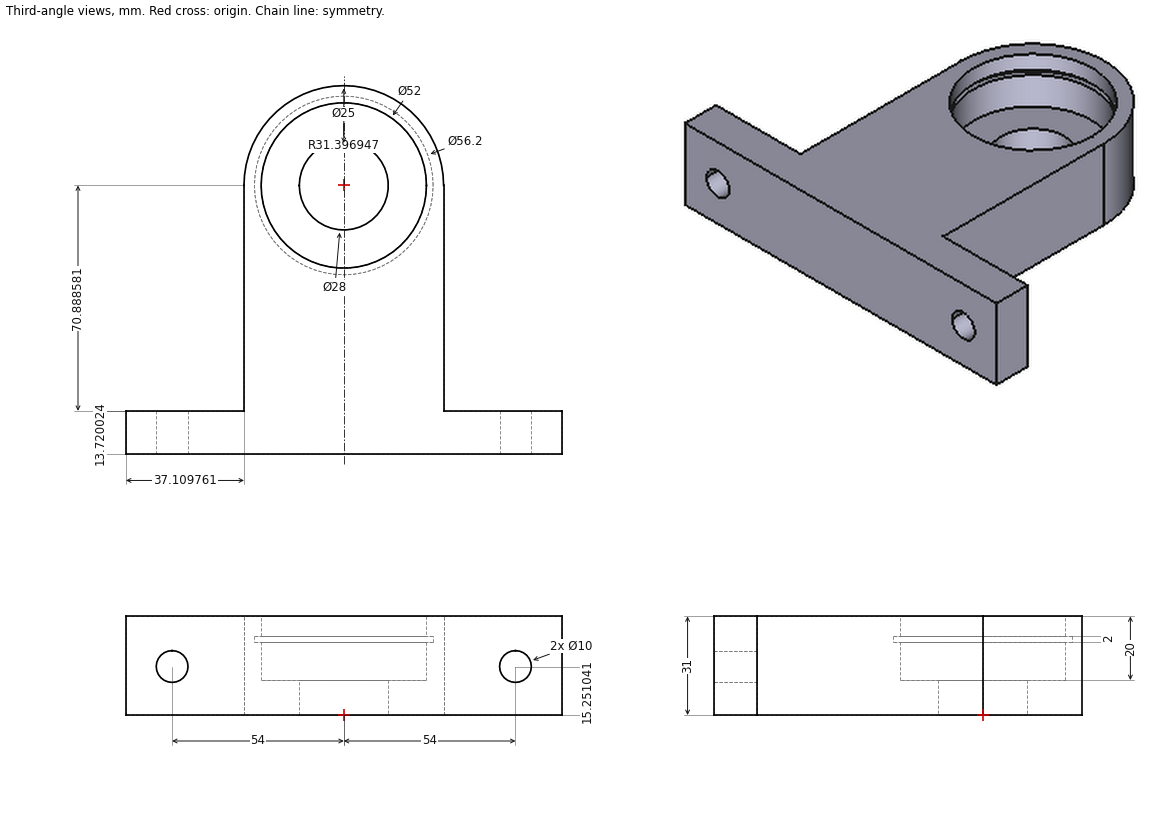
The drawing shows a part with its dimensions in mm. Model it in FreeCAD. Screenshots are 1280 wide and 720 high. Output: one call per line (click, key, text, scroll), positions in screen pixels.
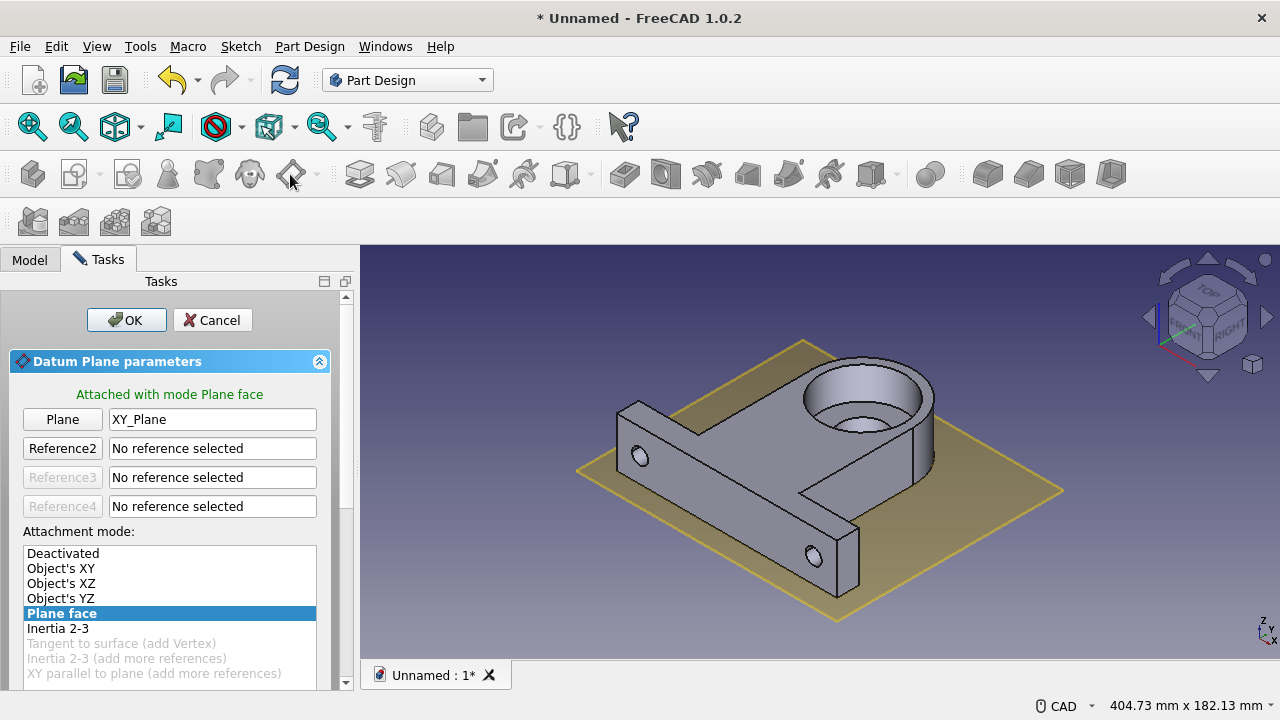
scroll(346, 490, down, 4)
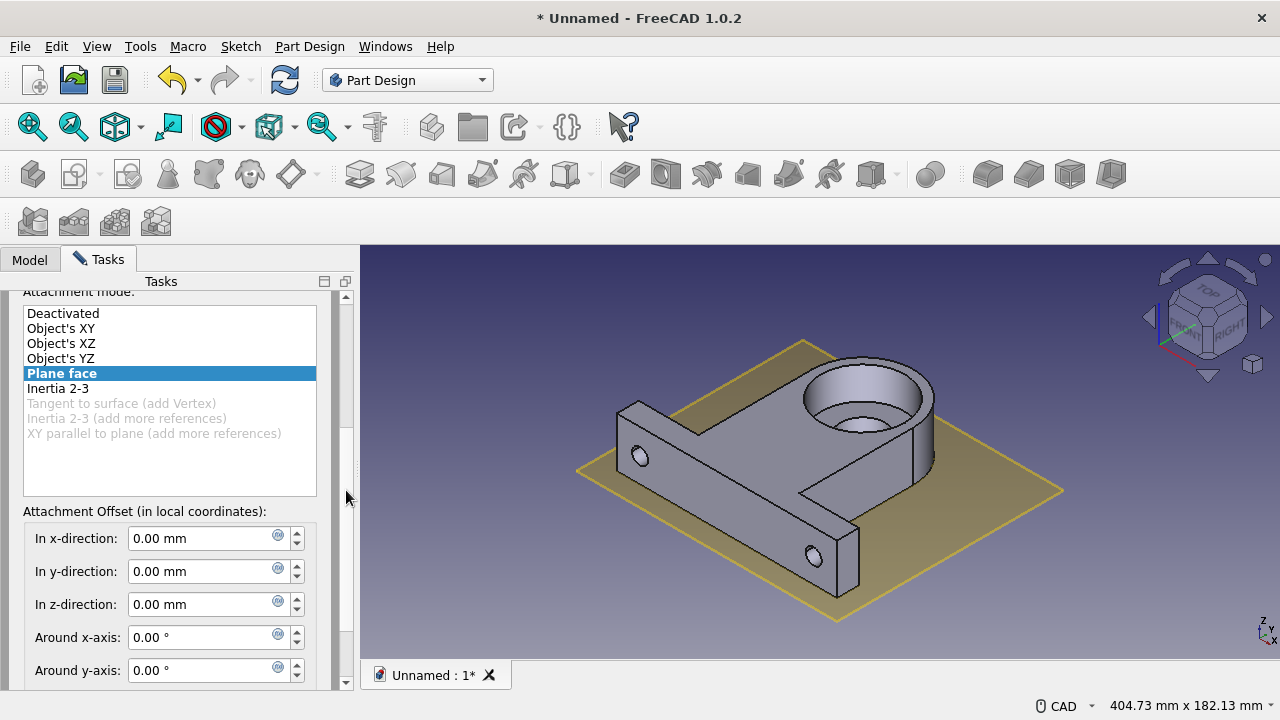
triple_click(210, 604)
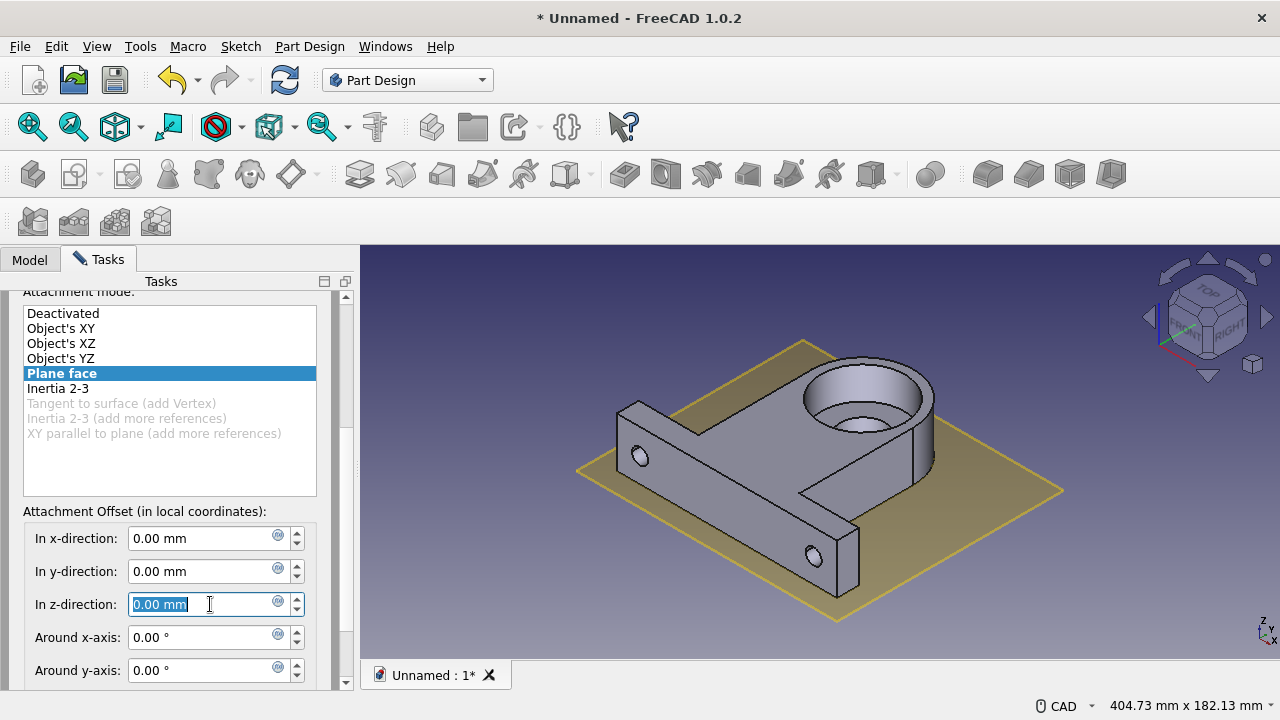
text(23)
key(Tab)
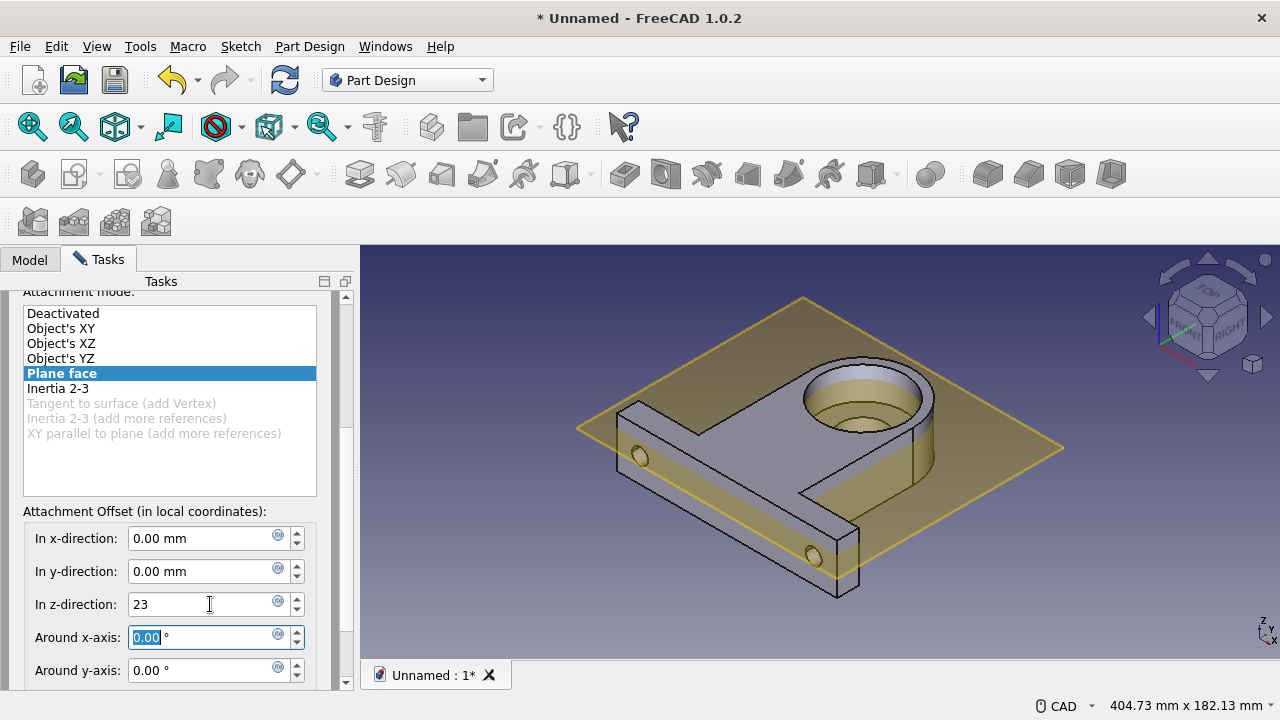
scroll(346, 490, up, 5)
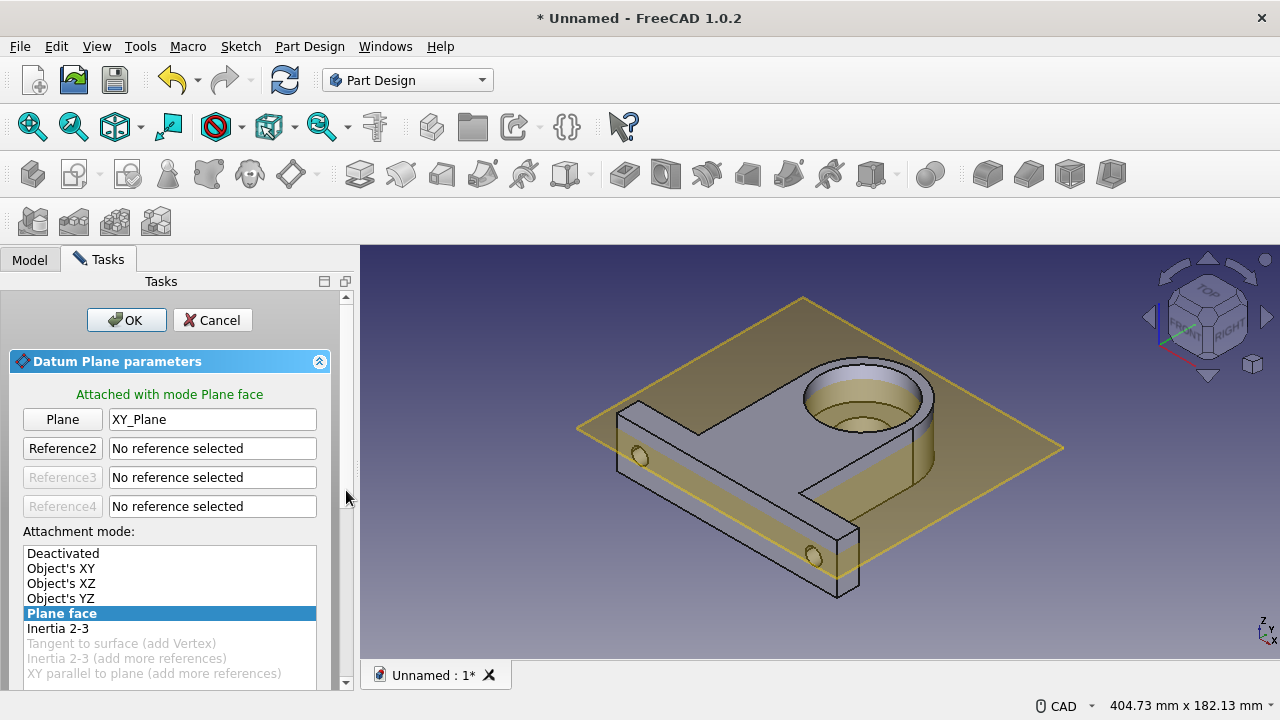
click(127, 320)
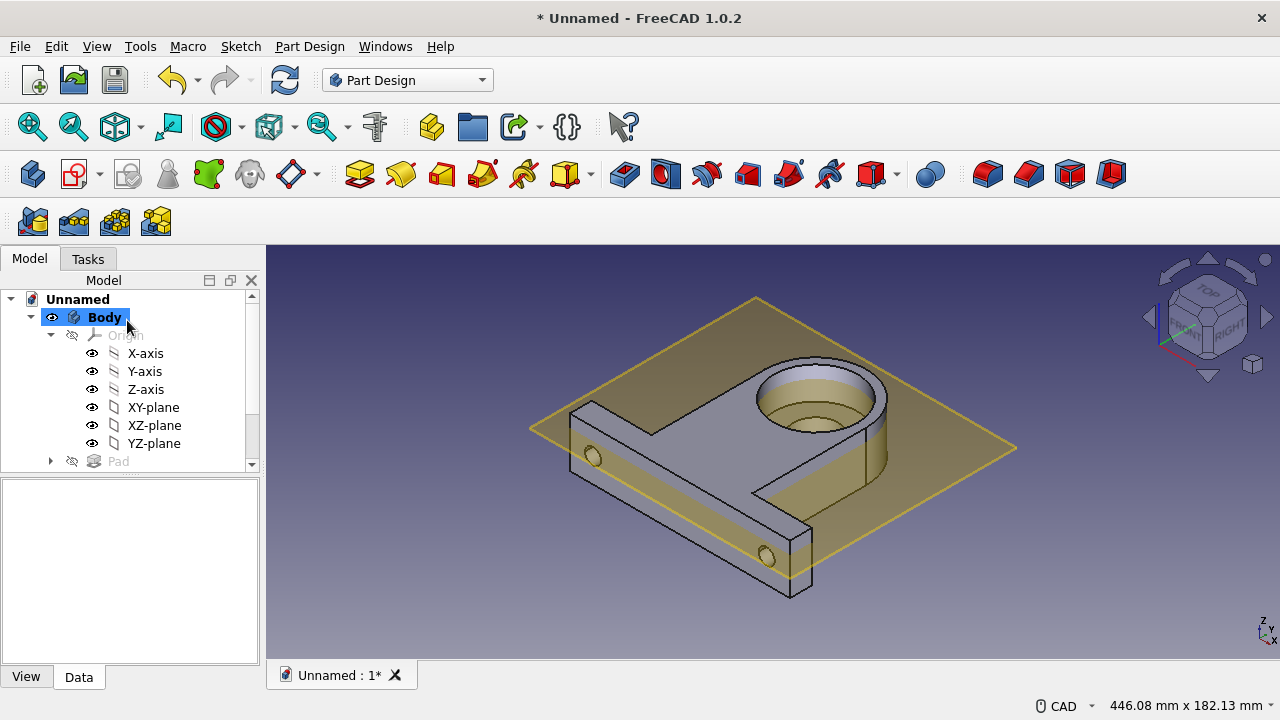
scroll(101, 385, down, 3)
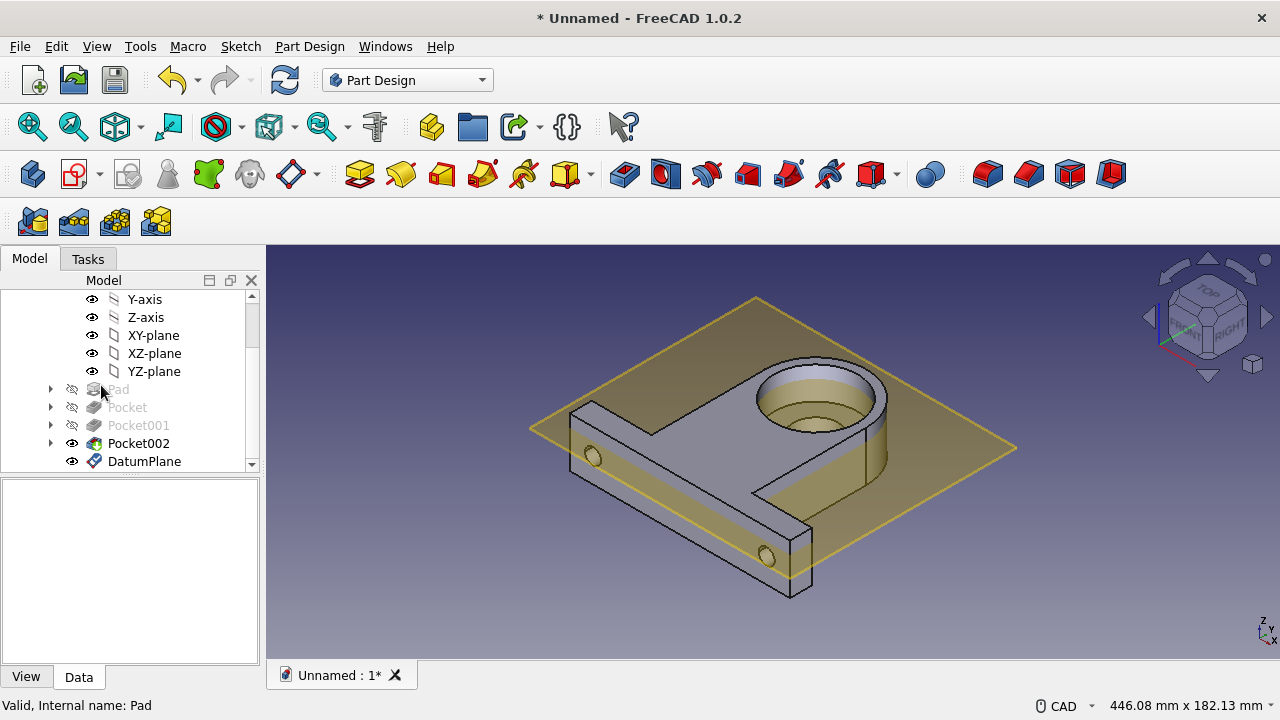
click(117, 461)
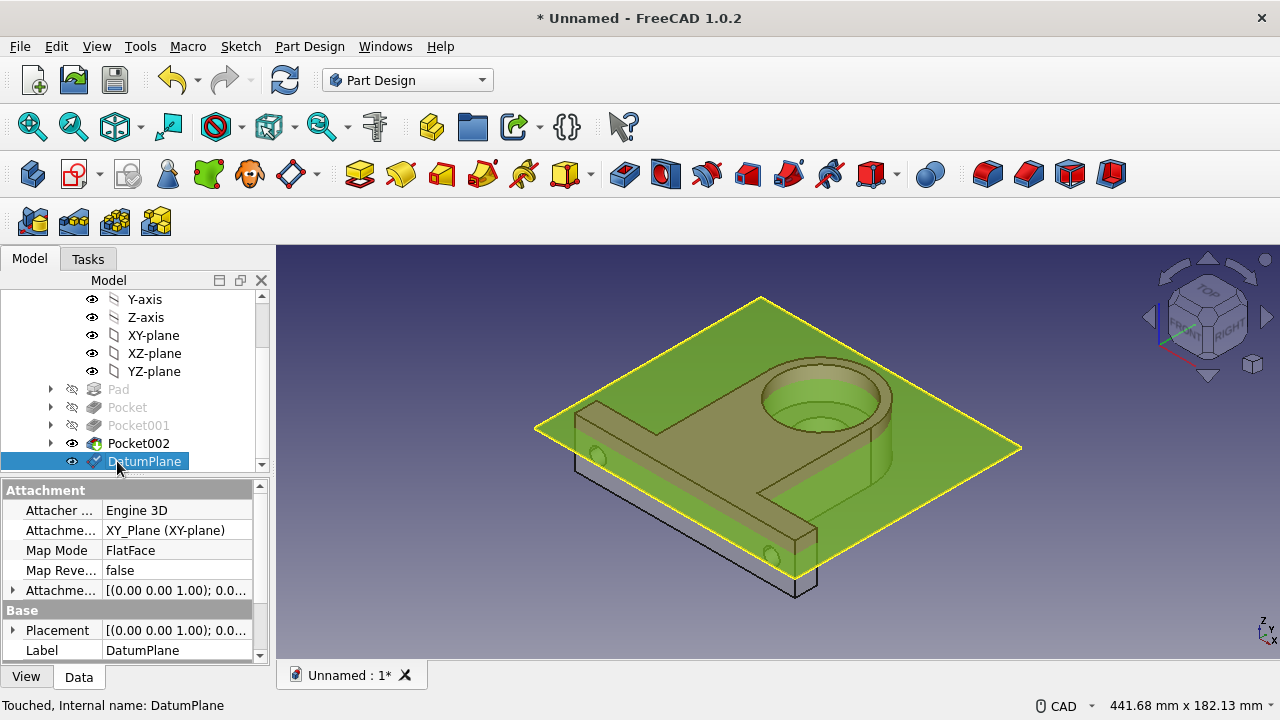
click(74, 174)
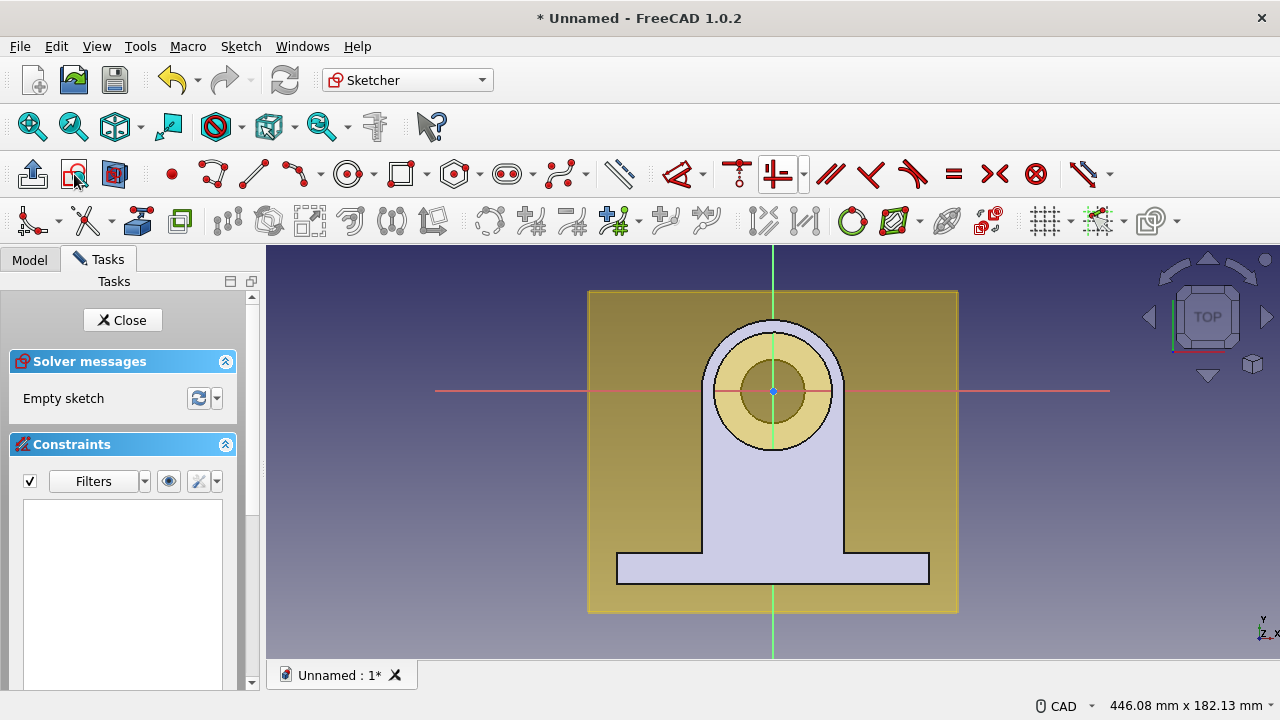
click(115, 174)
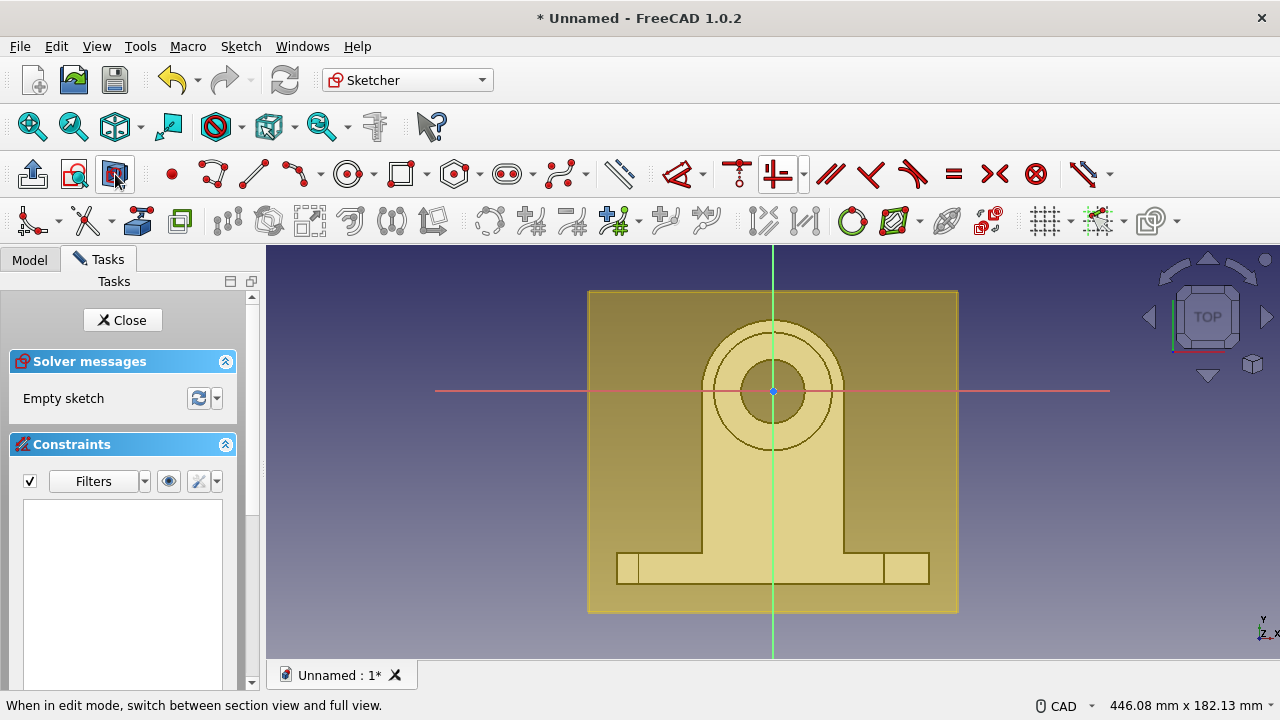
scroll(856, 318, up, 3)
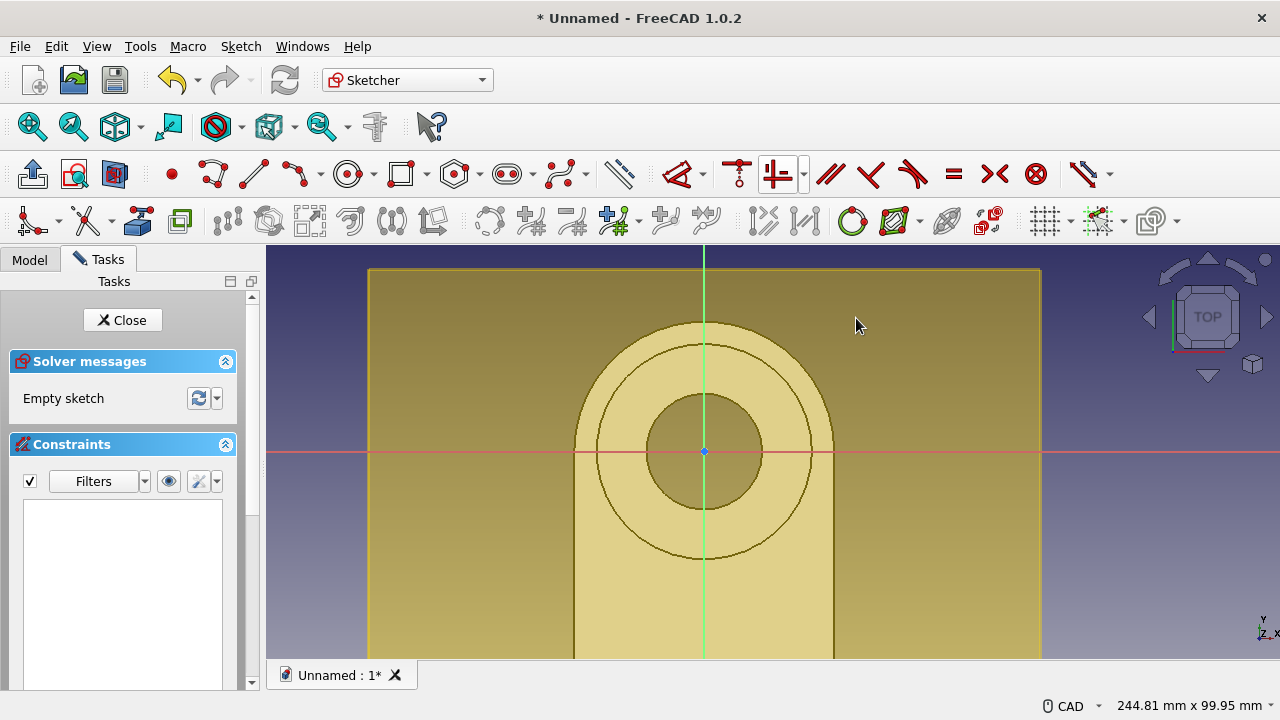
click(348, 174)